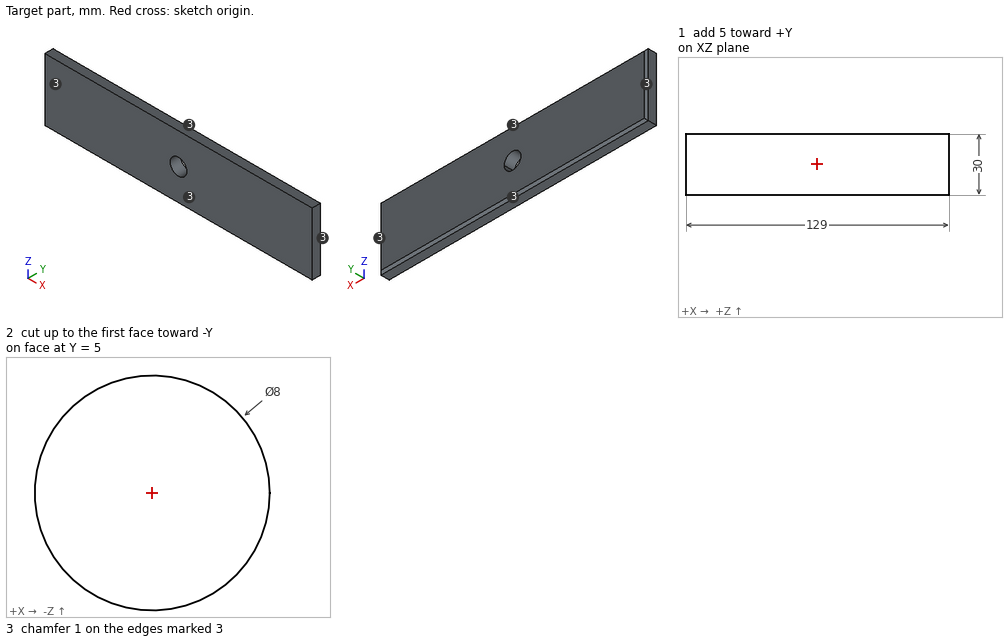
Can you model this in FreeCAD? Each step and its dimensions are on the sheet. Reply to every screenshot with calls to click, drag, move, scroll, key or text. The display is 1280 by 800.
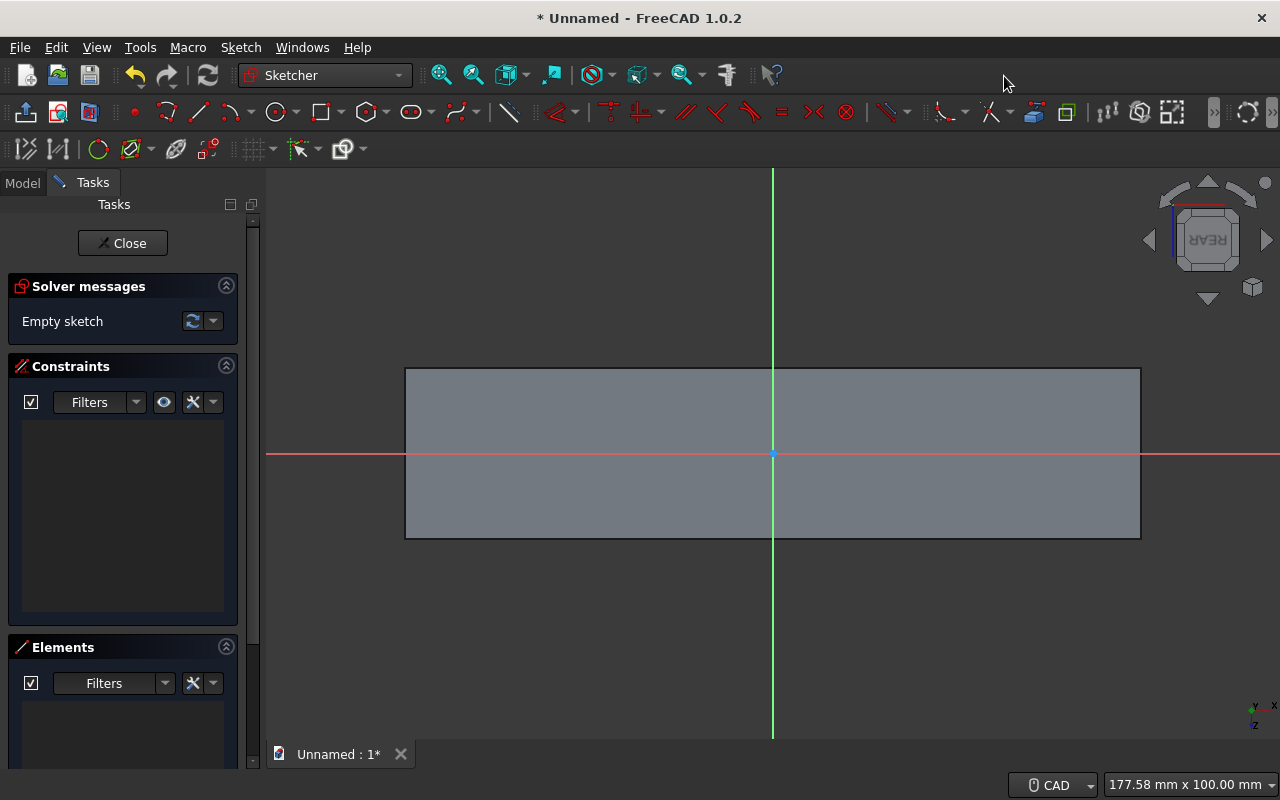
scroll(784, 454, up, 10)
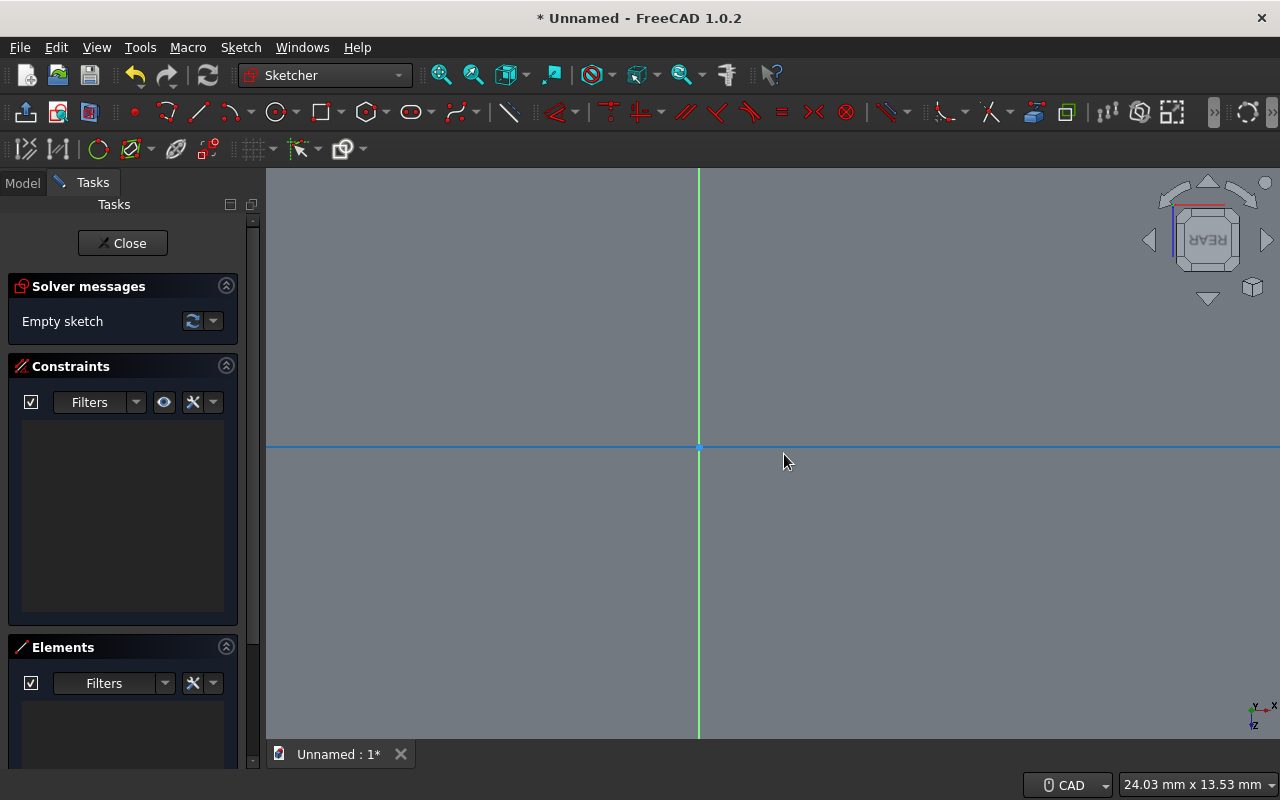
key(g)
key(c)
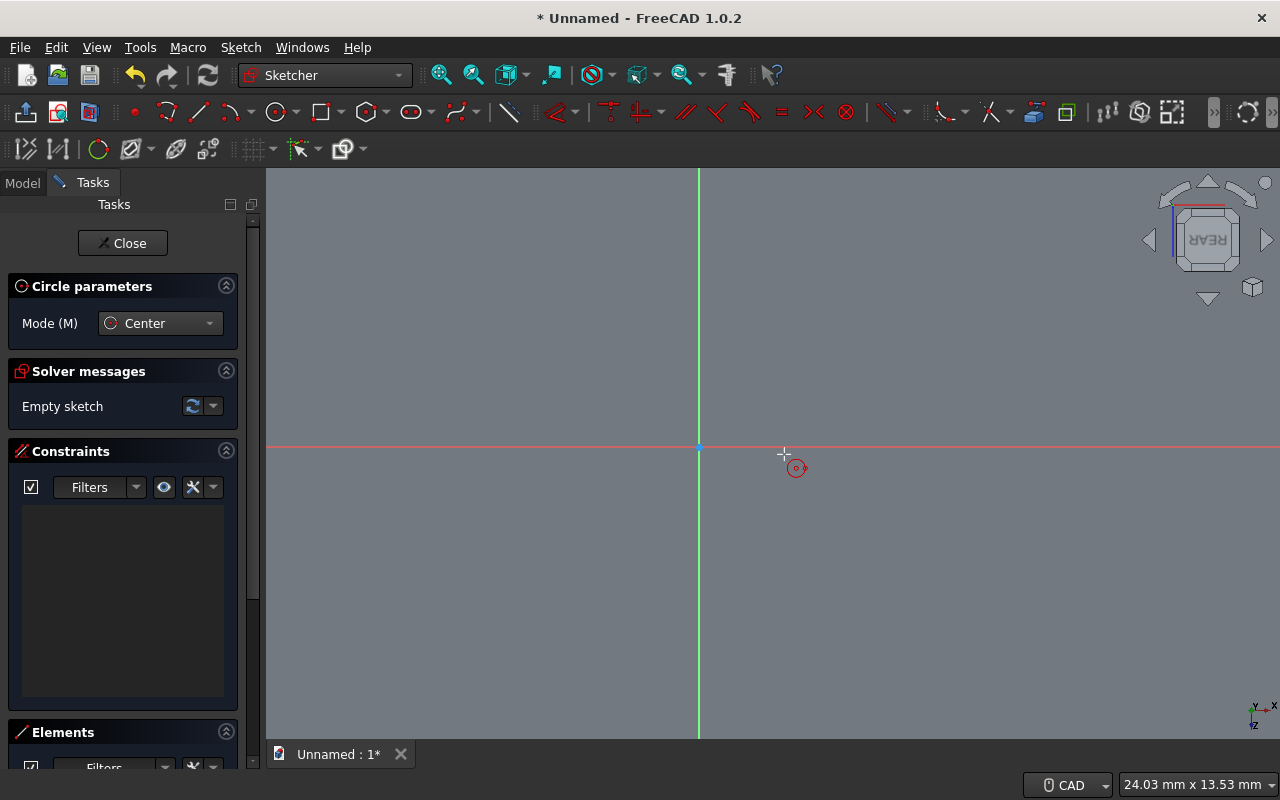
click(699, 447)
click(819, 328)
key(Escape)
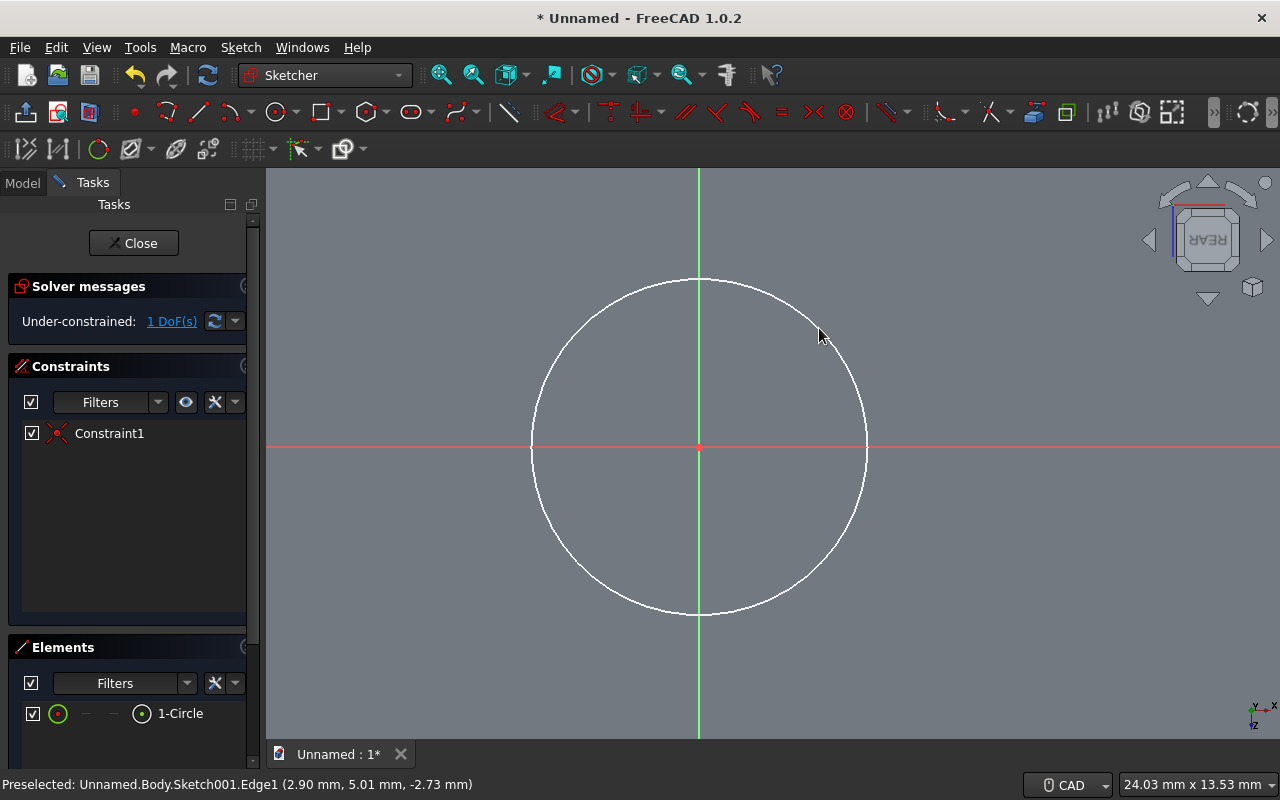
key(d)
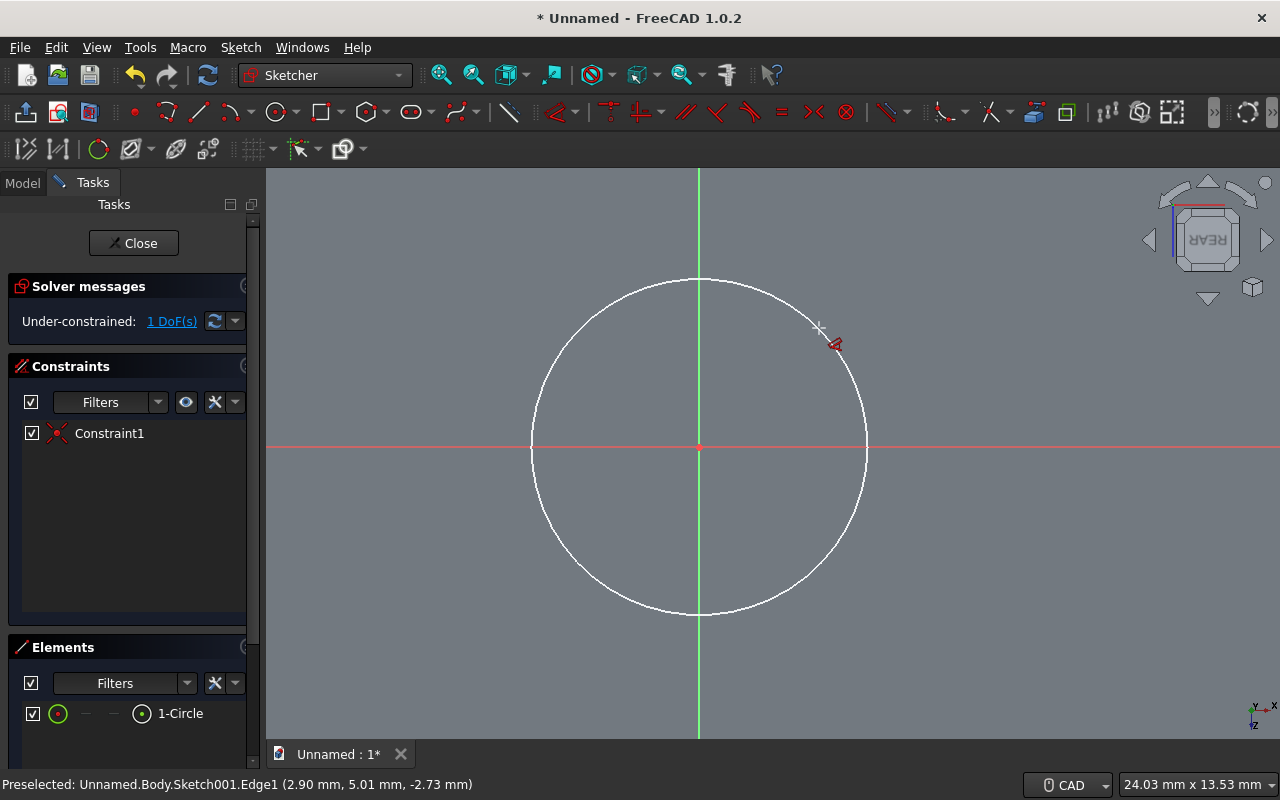
click(818, 328)
click(841, 305)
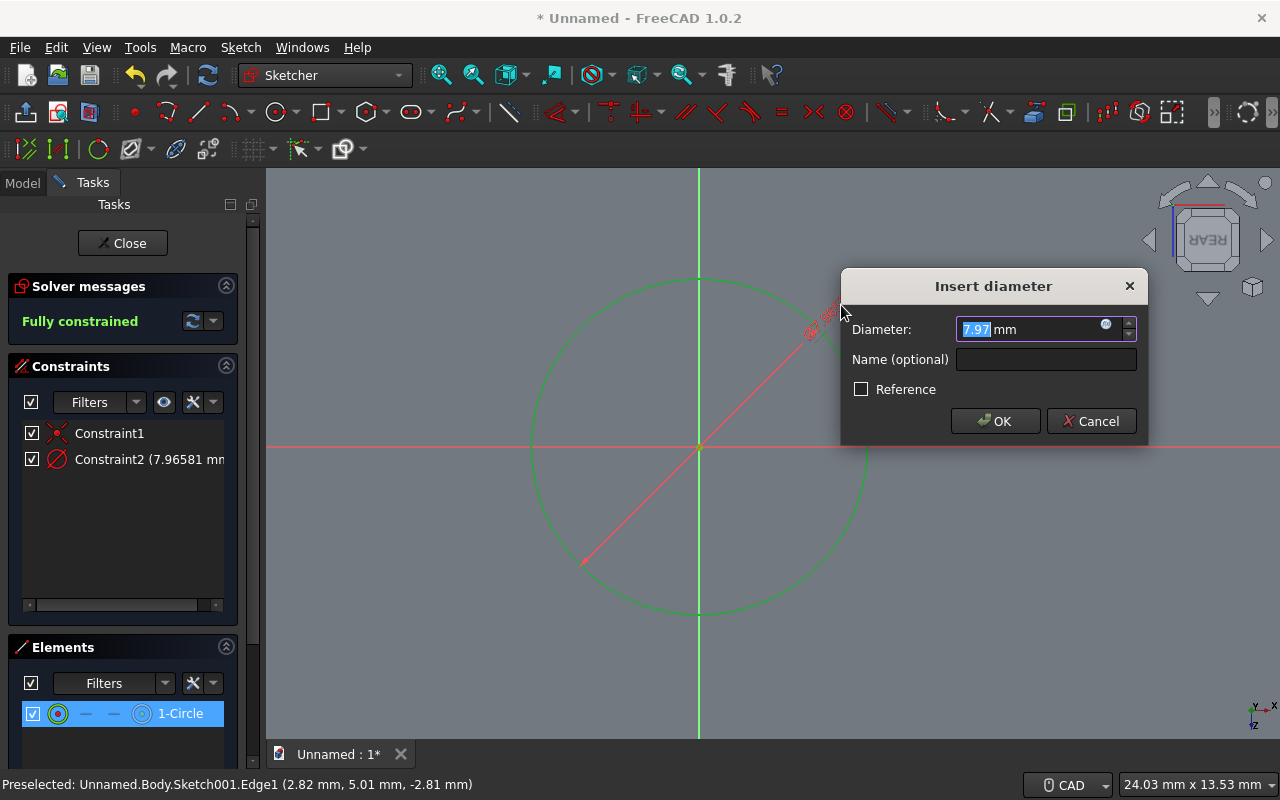
text(8)
key(Return)
key(Escape)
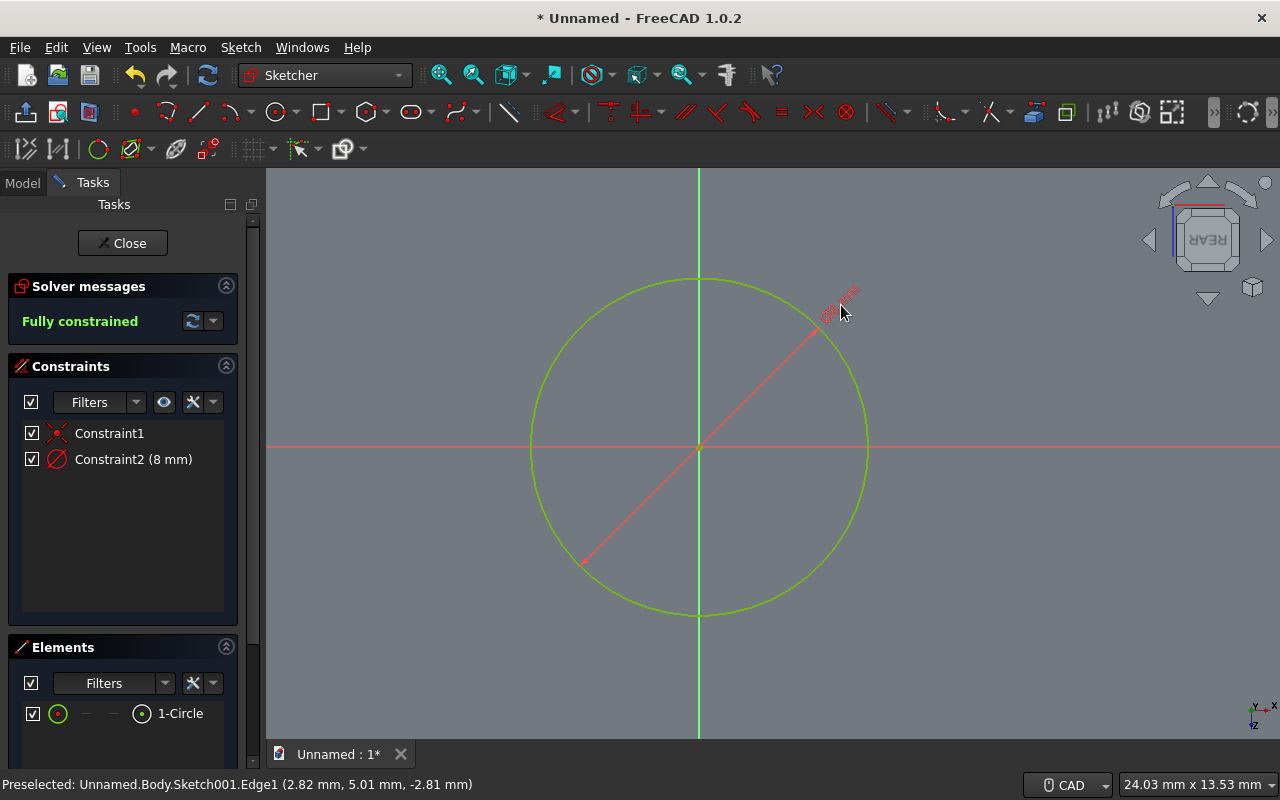
click(123, 243)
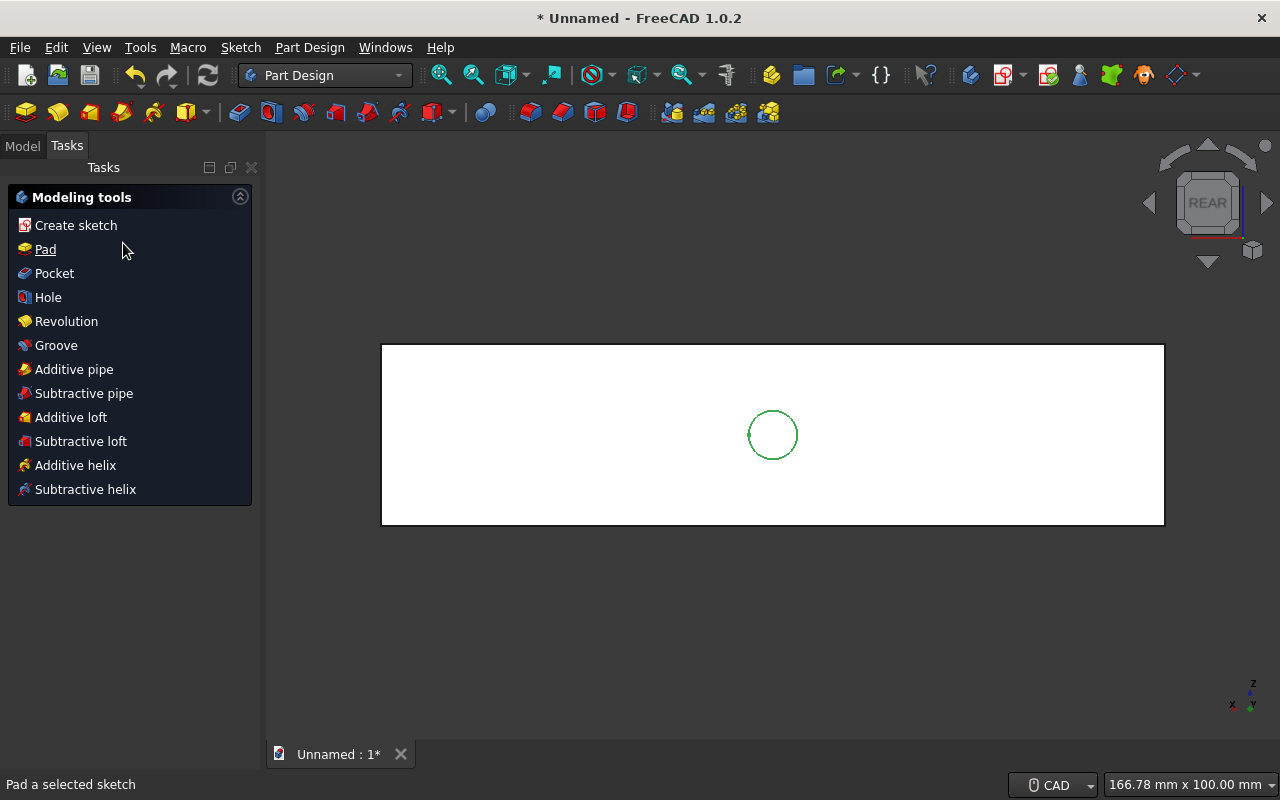
click(240, 112)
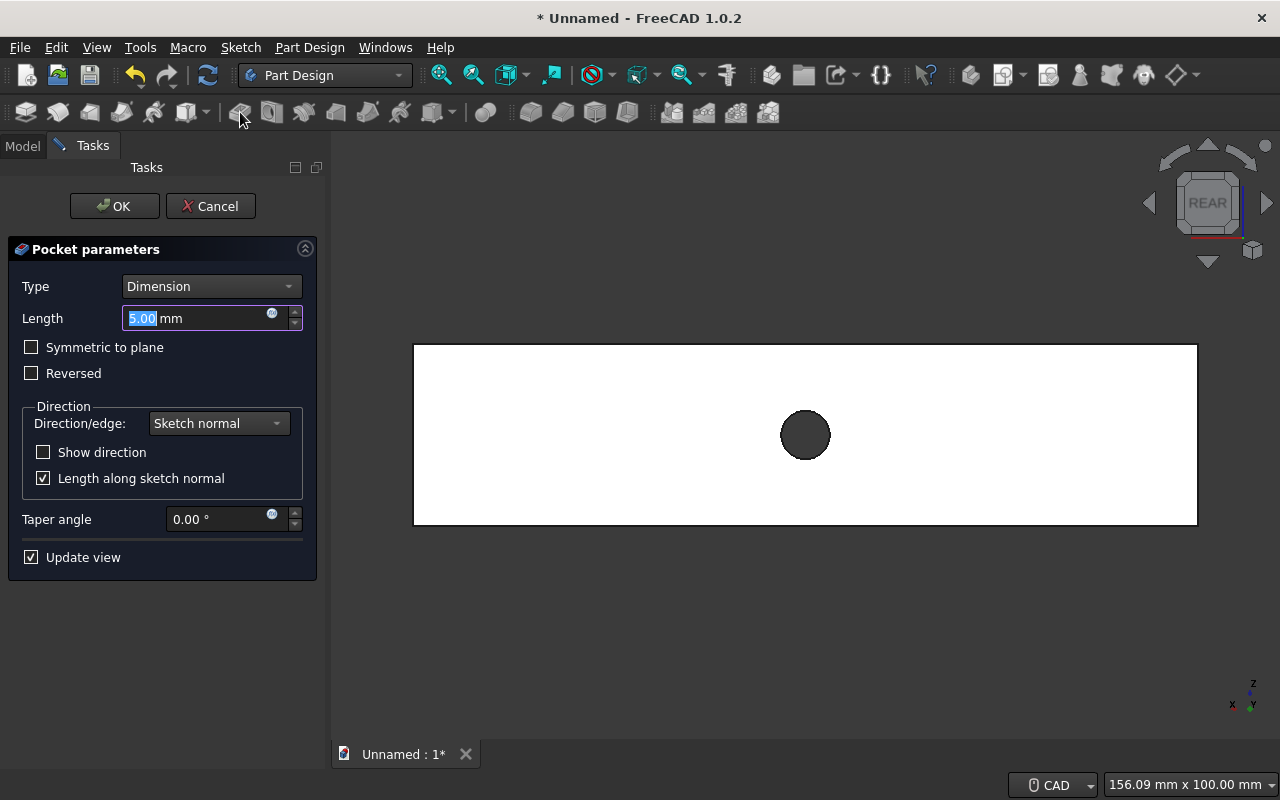
click(212, 286)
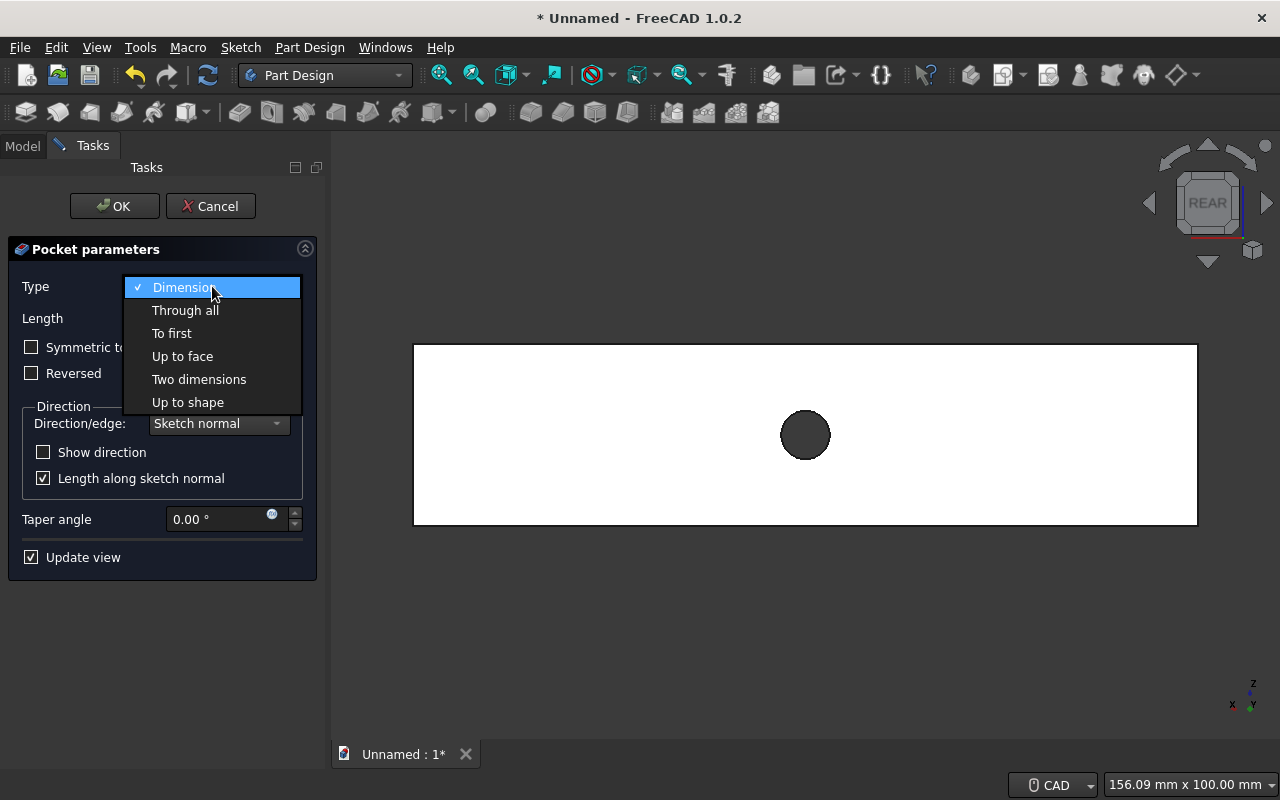
click(212, 334)